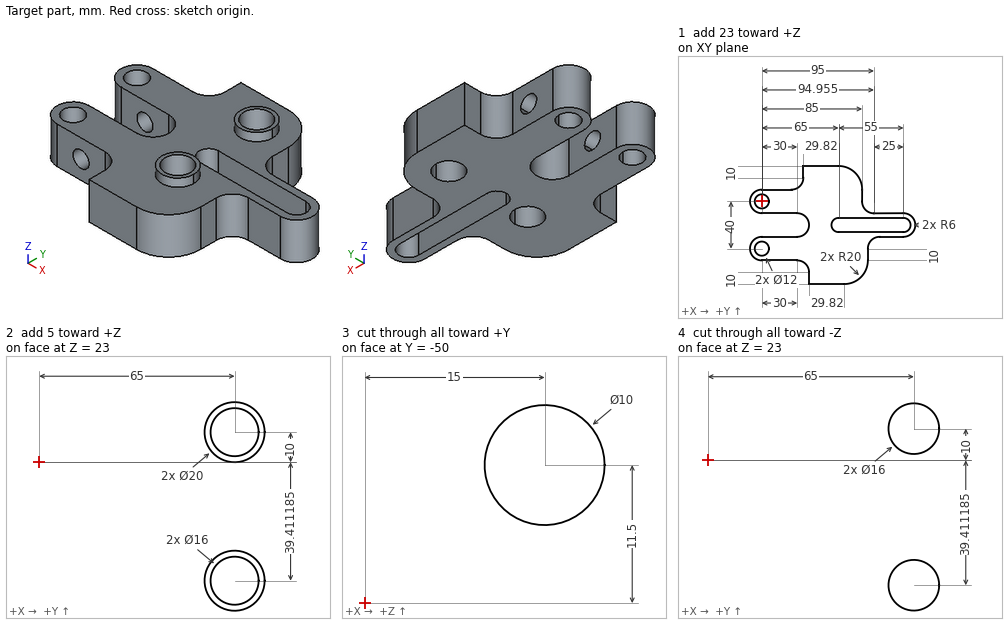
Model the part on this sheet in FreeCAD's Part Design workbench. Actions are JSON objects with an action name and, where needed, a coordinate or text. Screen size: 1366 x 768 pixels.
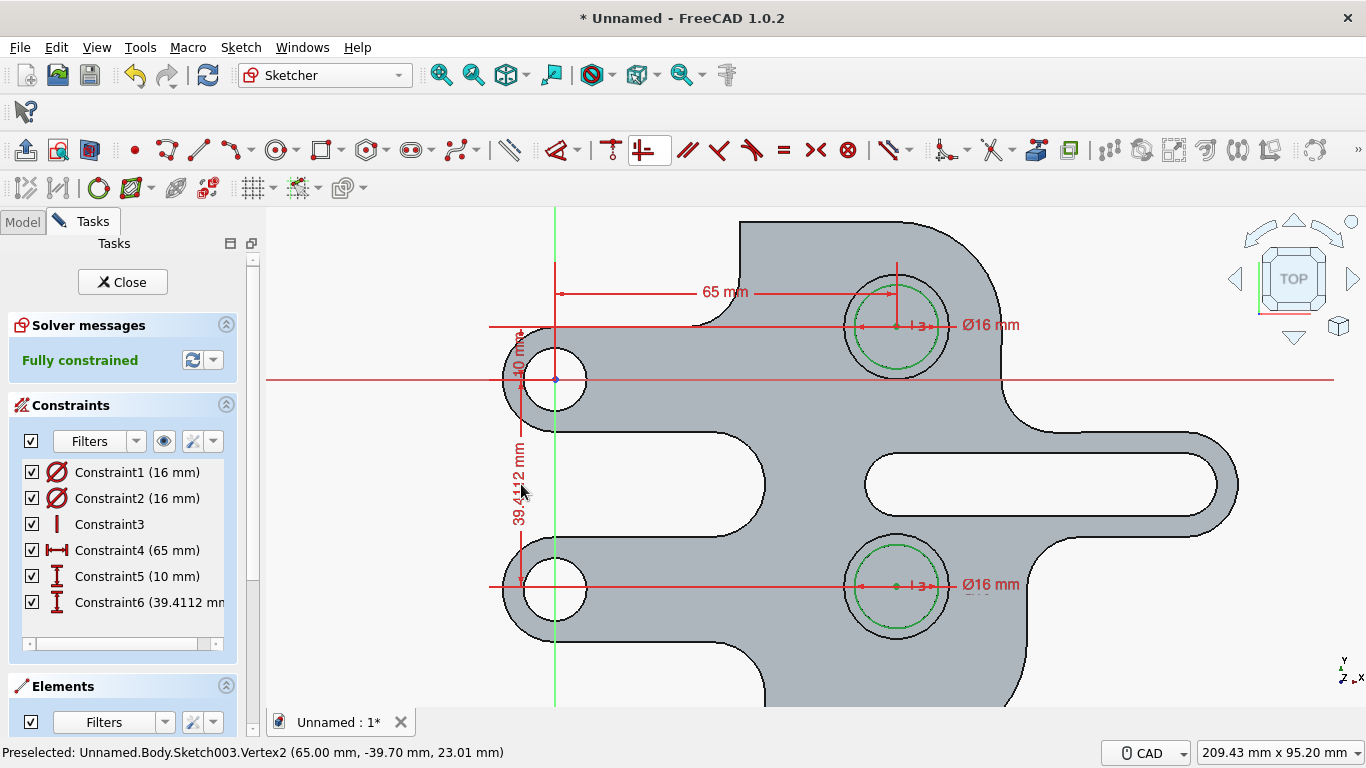
{"action": "left_click", "coordinate": [123, 282]}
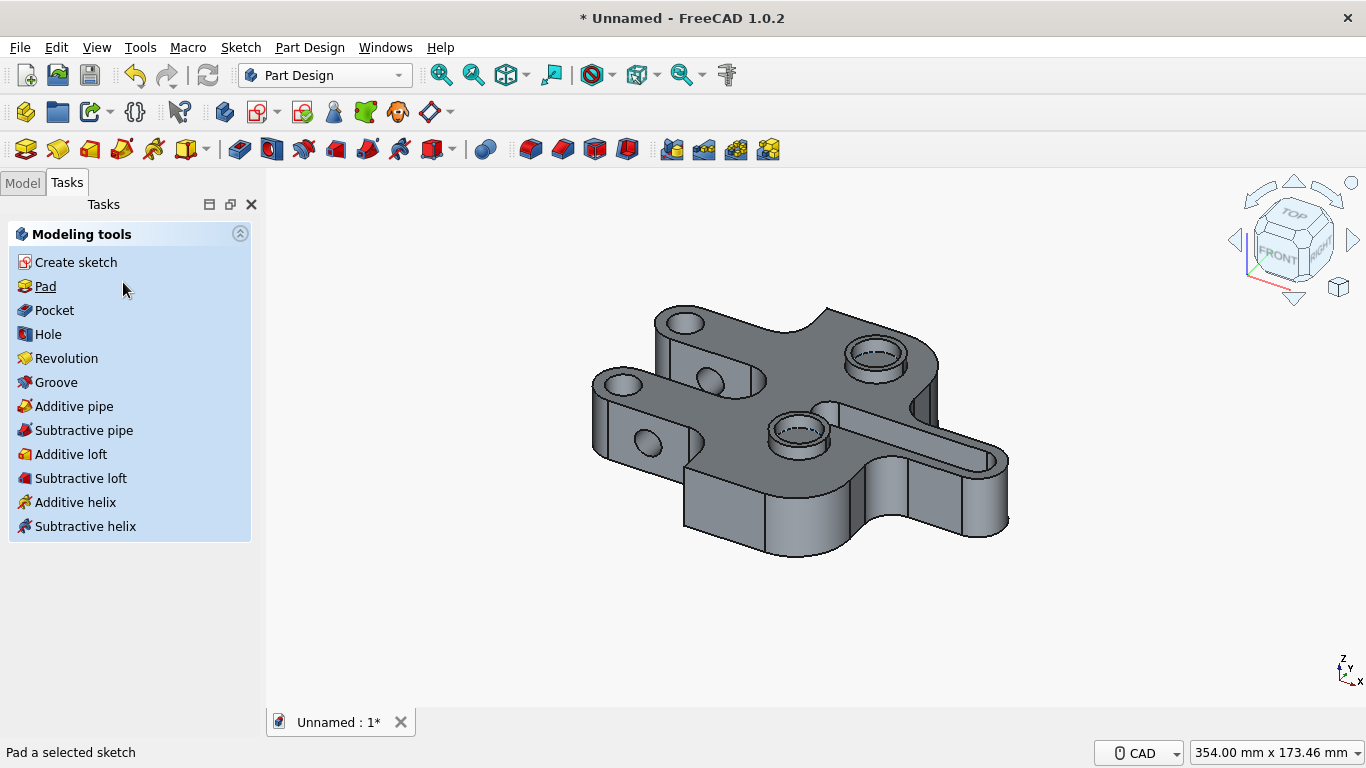
{"action": "left_click", "coordinate": [240, 150]}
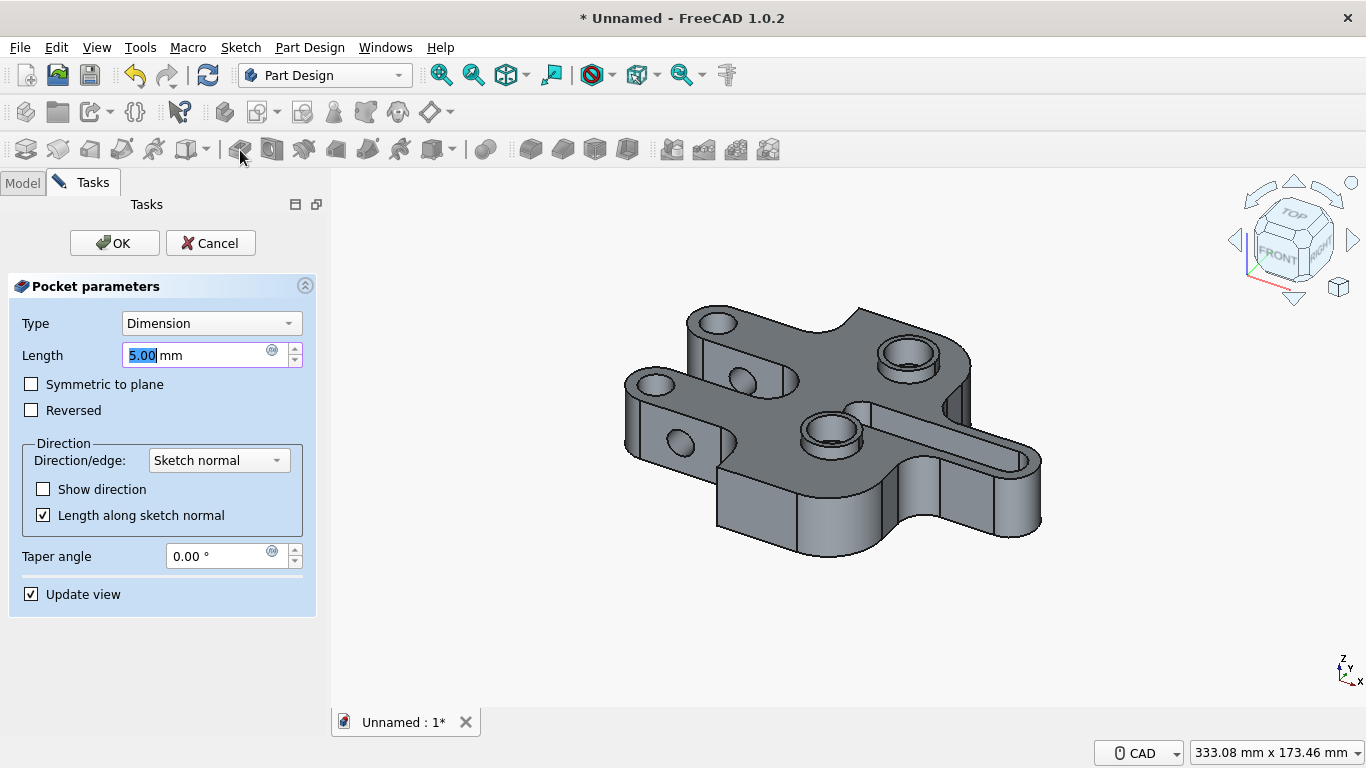
{"action": "left_click", "coordinate": [212, 324]}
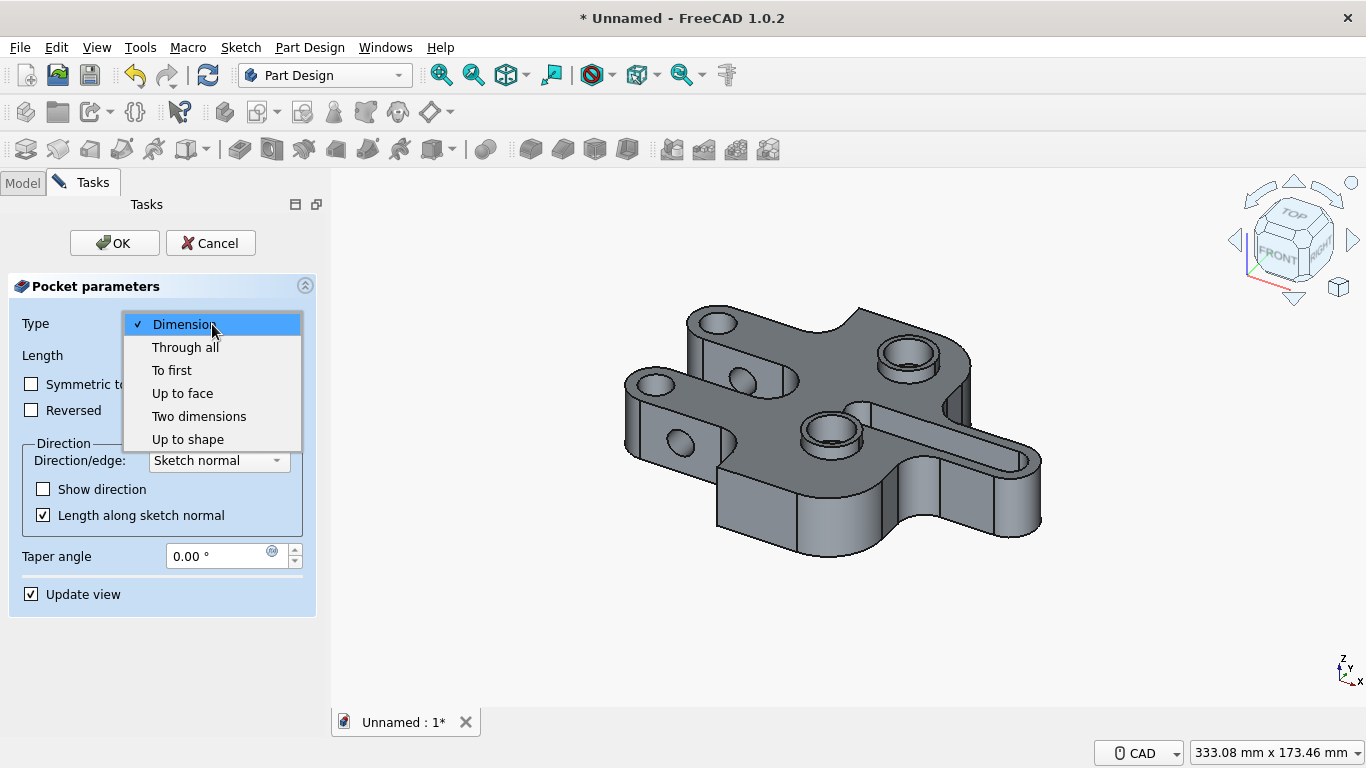
{"action": "left_click", "coordinate": [212, 348]}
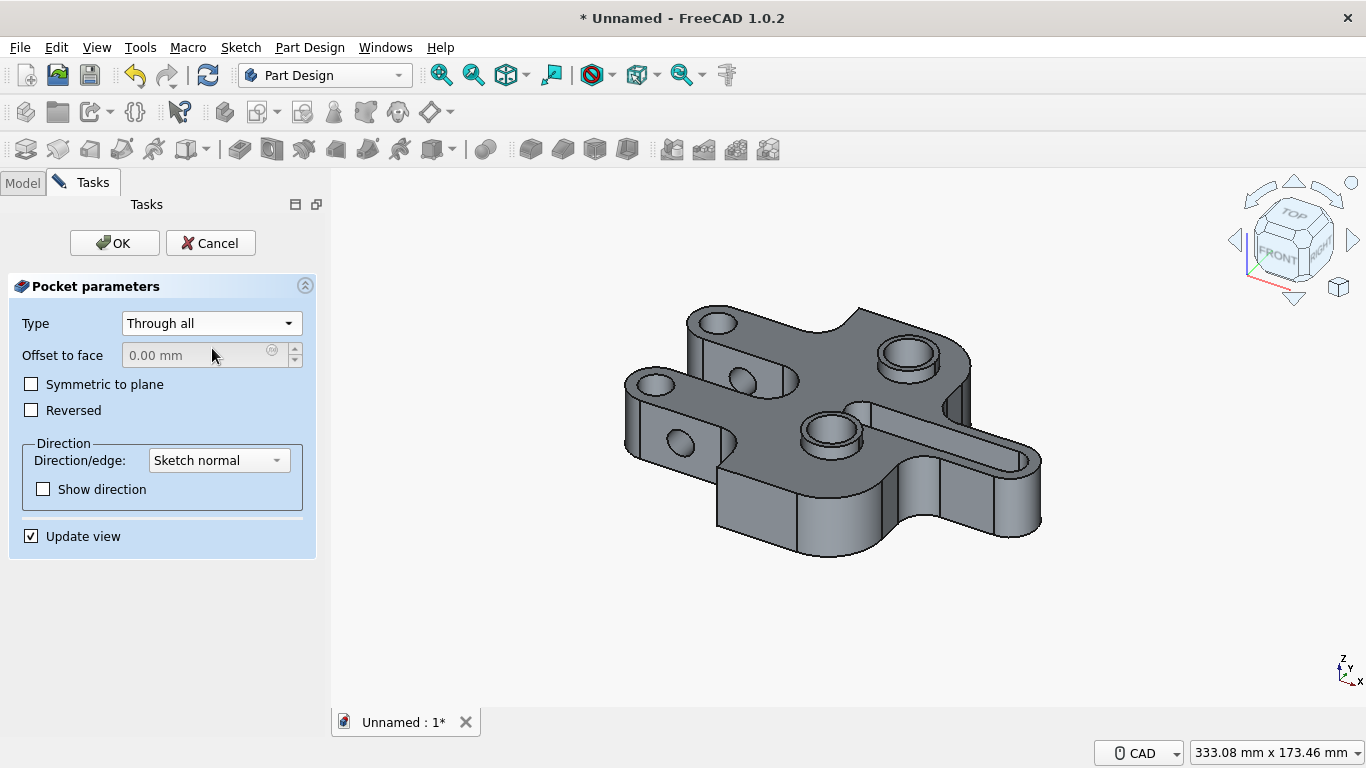
{"action": "left_click", "coordinate": [115, 243]}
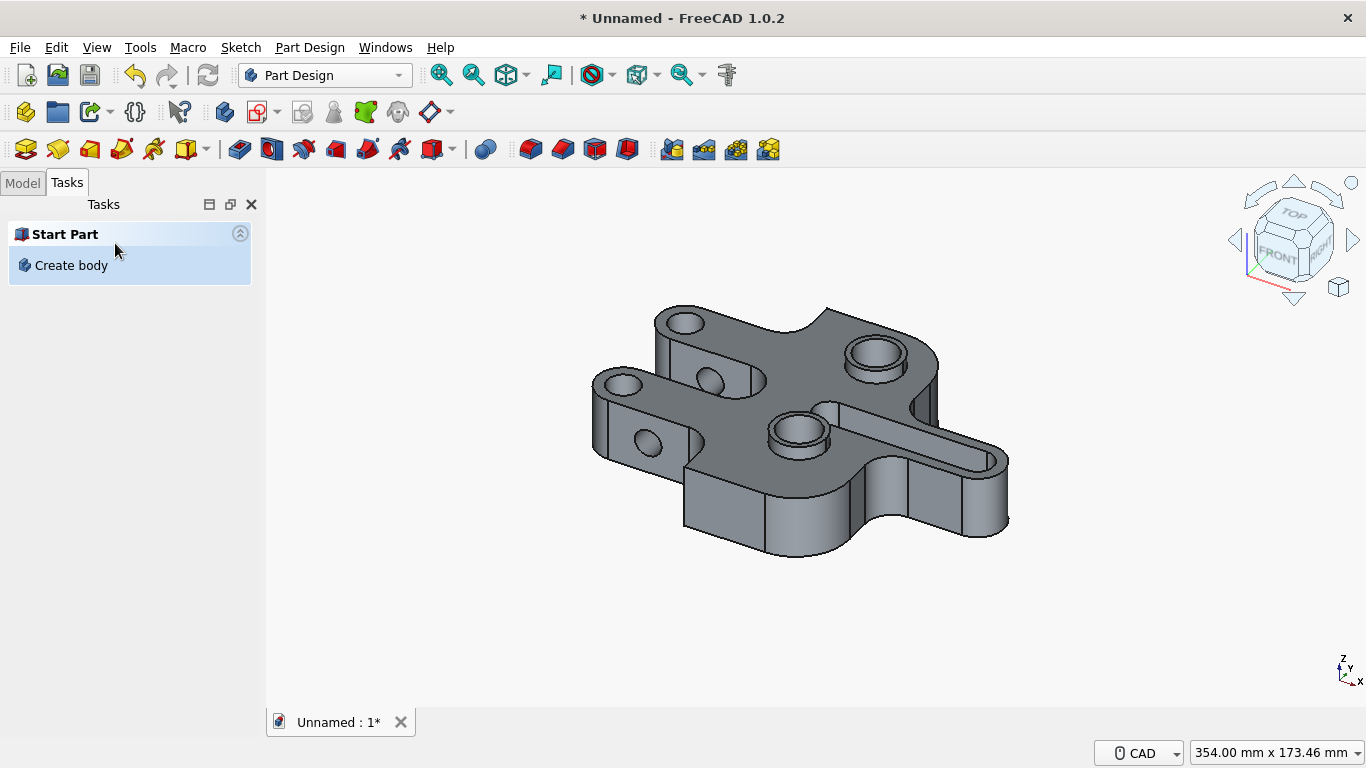
{"action": "key", "text": "0"}